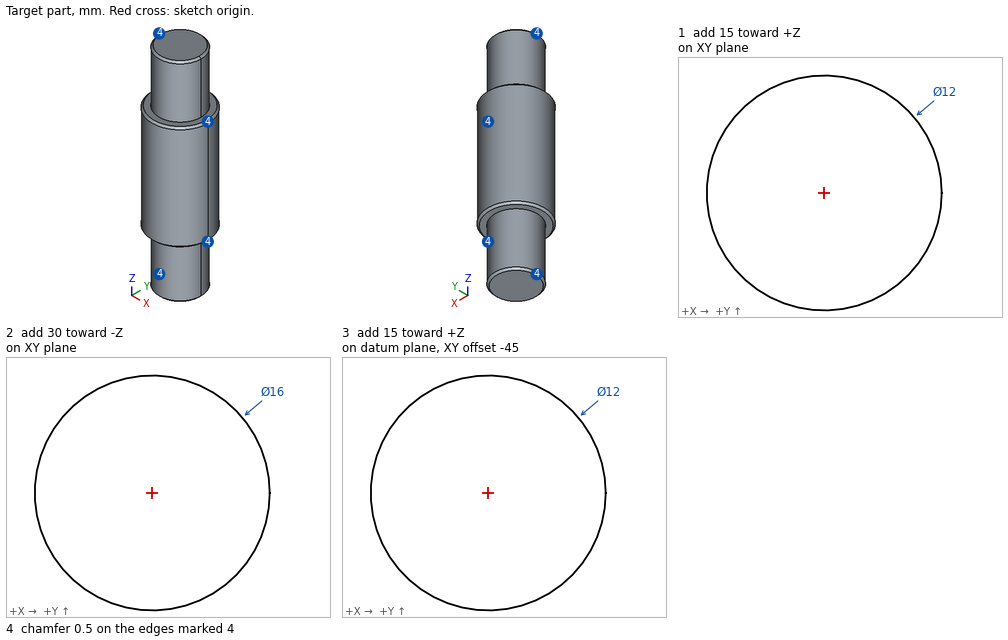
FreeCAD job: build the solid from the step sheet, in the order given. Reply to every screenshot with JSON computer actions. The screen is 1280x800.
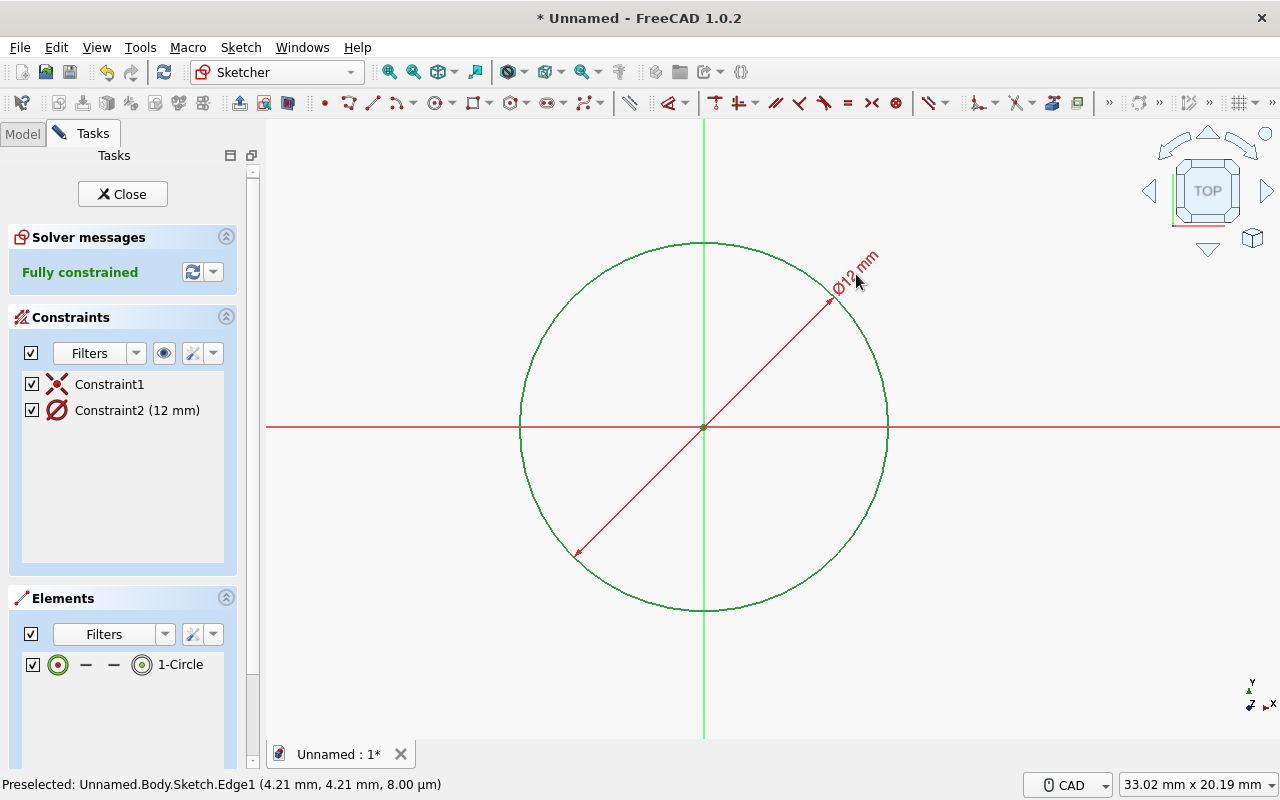
{"action": "left_click", "coordinate": [123, 194]}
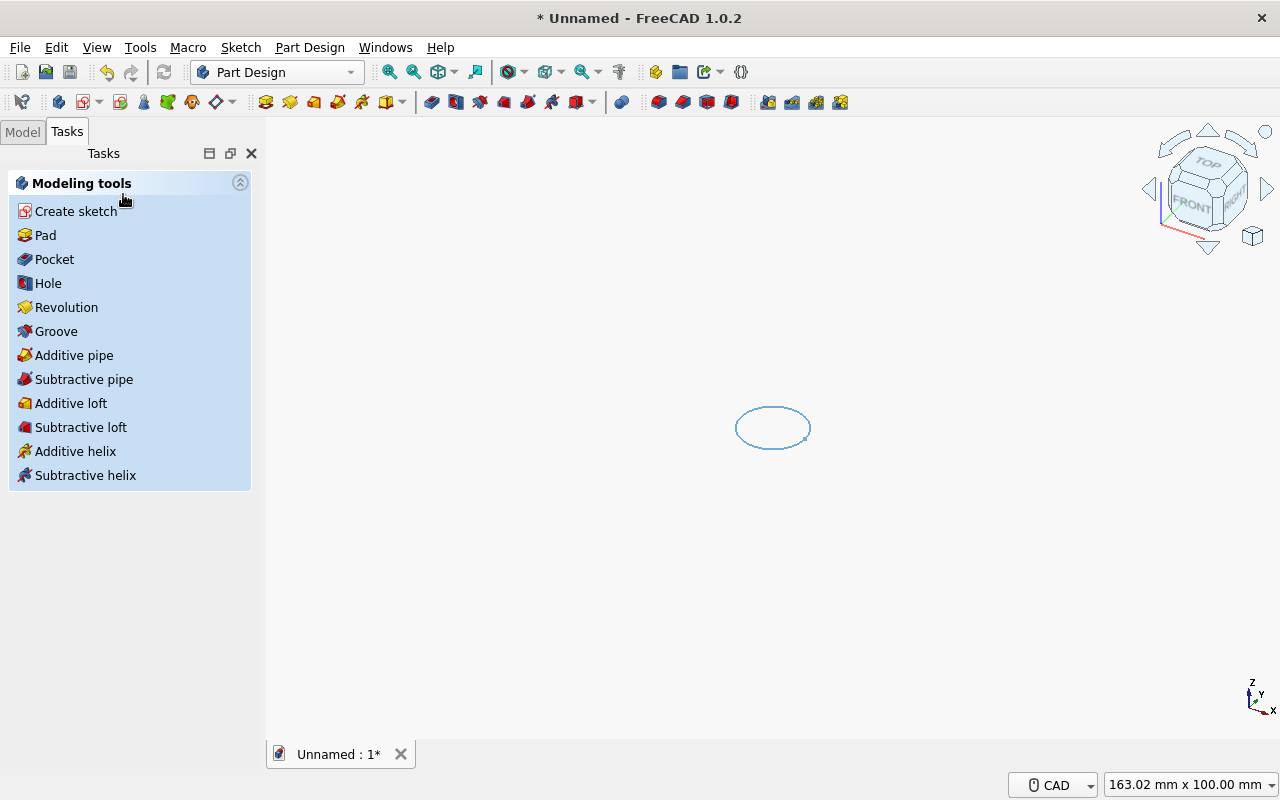
{"action": "left_click", "coordinate": [266, 102]}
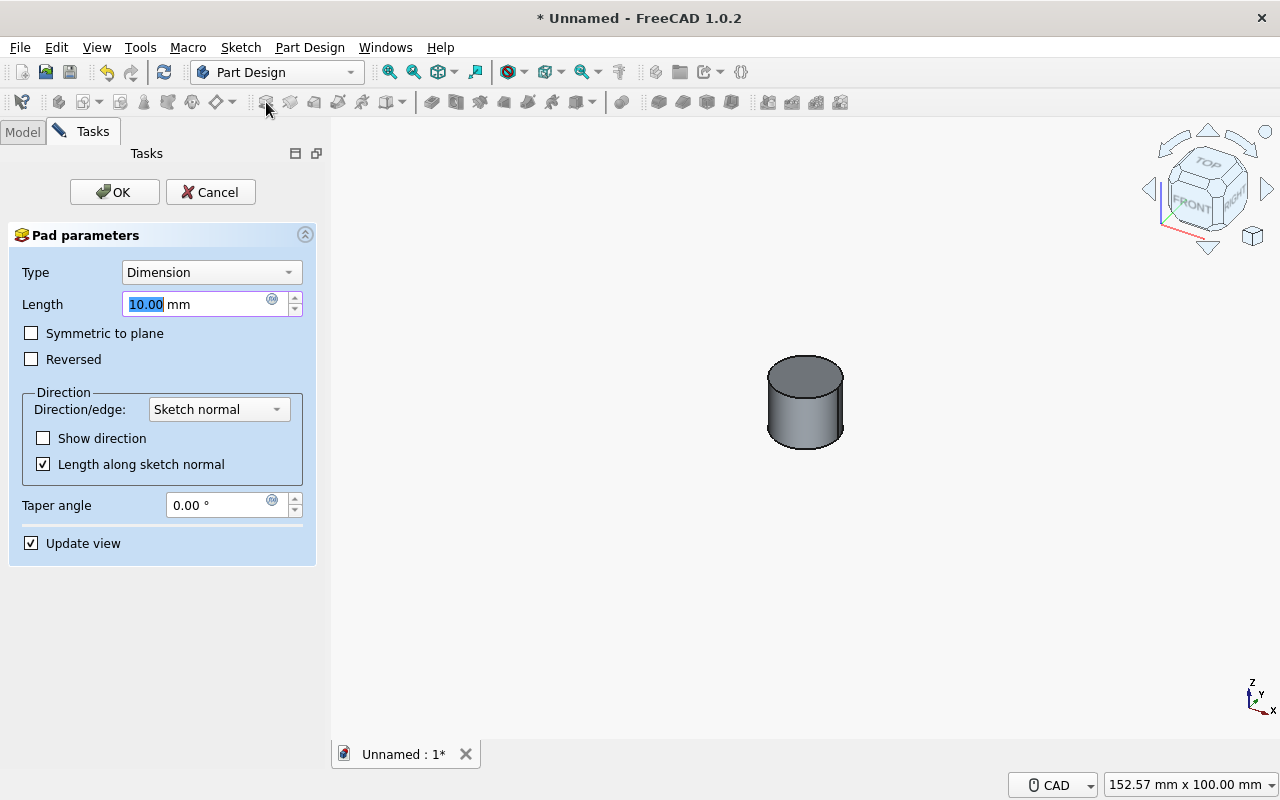
{"action": "type", "text": "15"}
{"action": "key", "text": "Tab"}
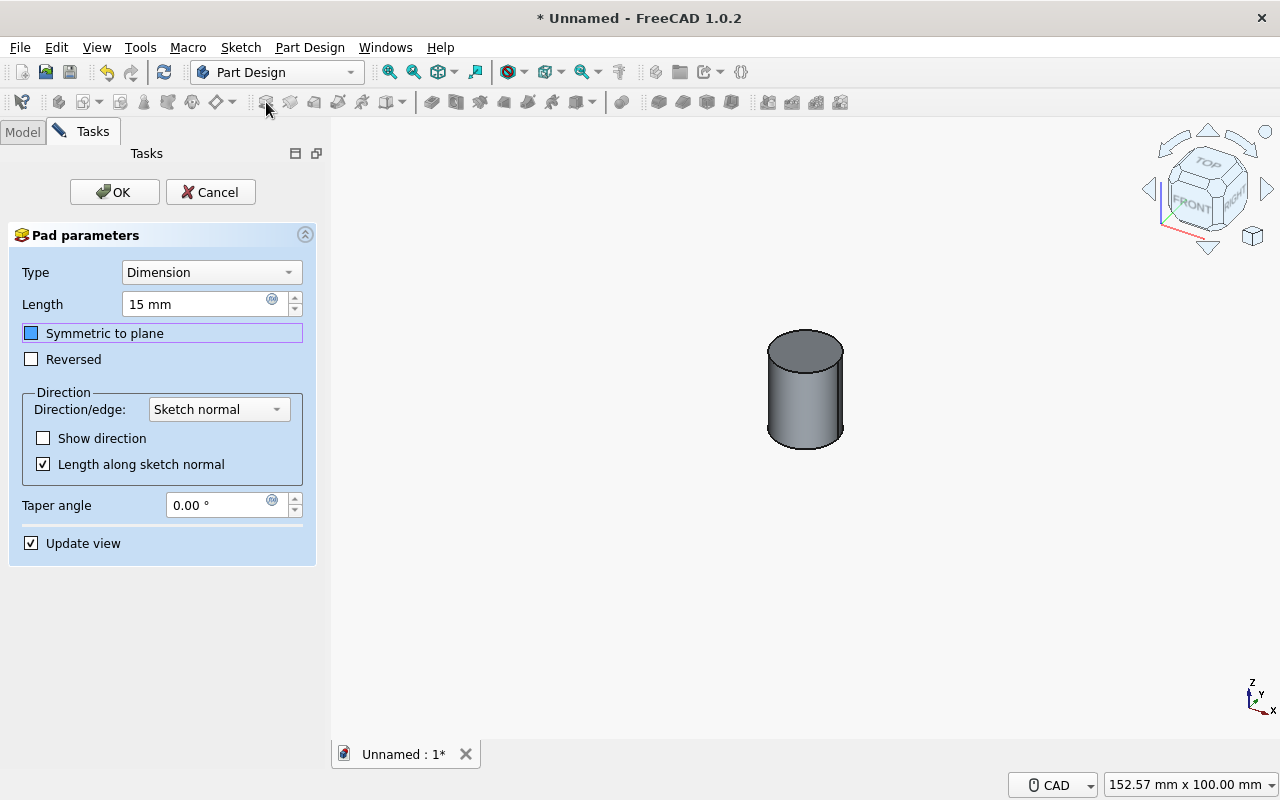
{"action": "left_click", "coordinate": [115, 192]}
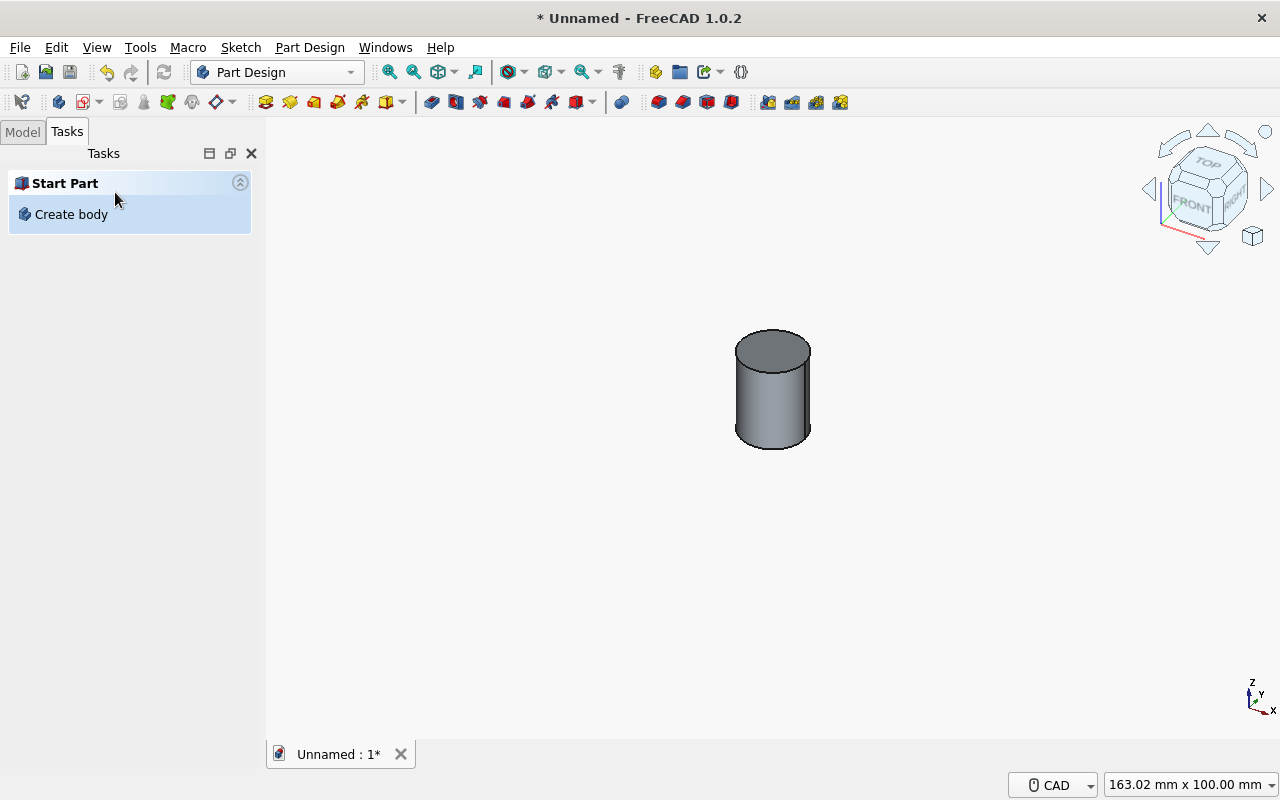
{"action": "left_click", "coordinate": [390, 72]}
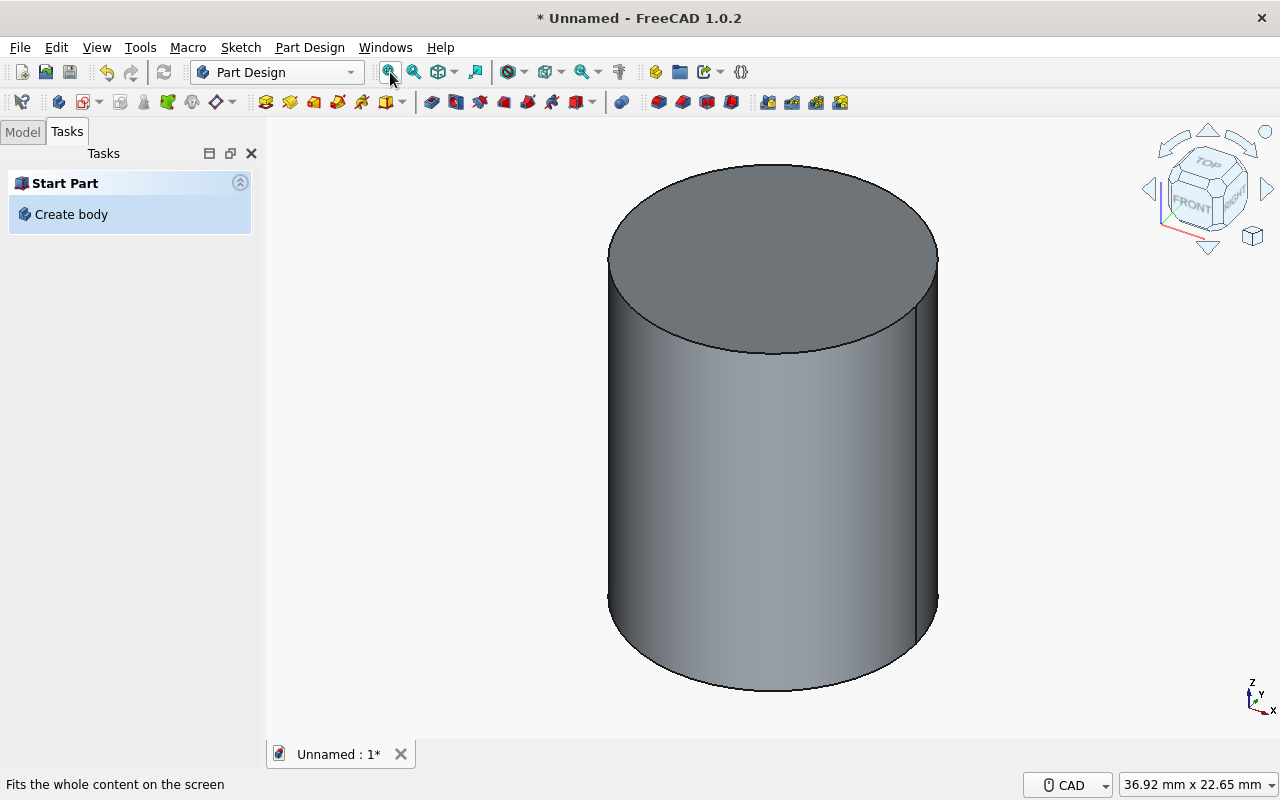
{"action": "left_click", "coordinate": [84, 102]}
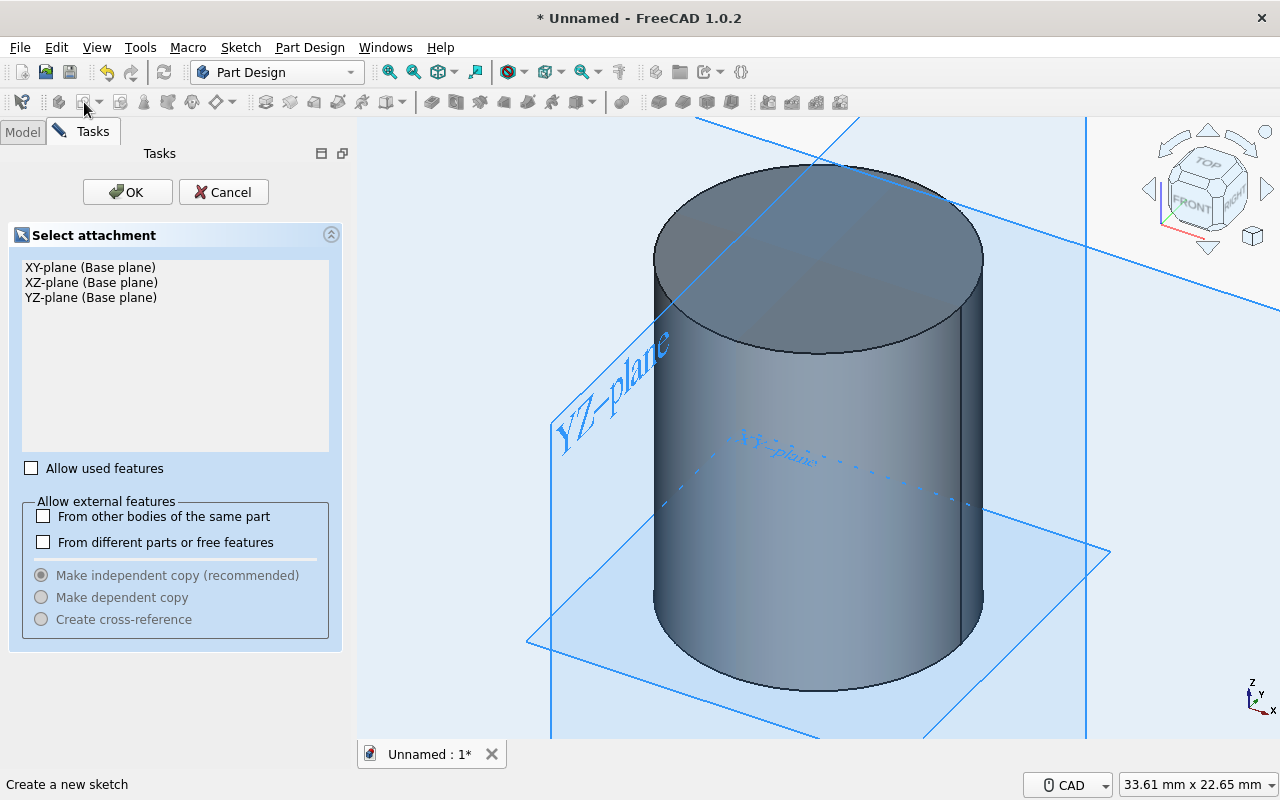
{"action": "left_click", "coordinate": [82, 268]}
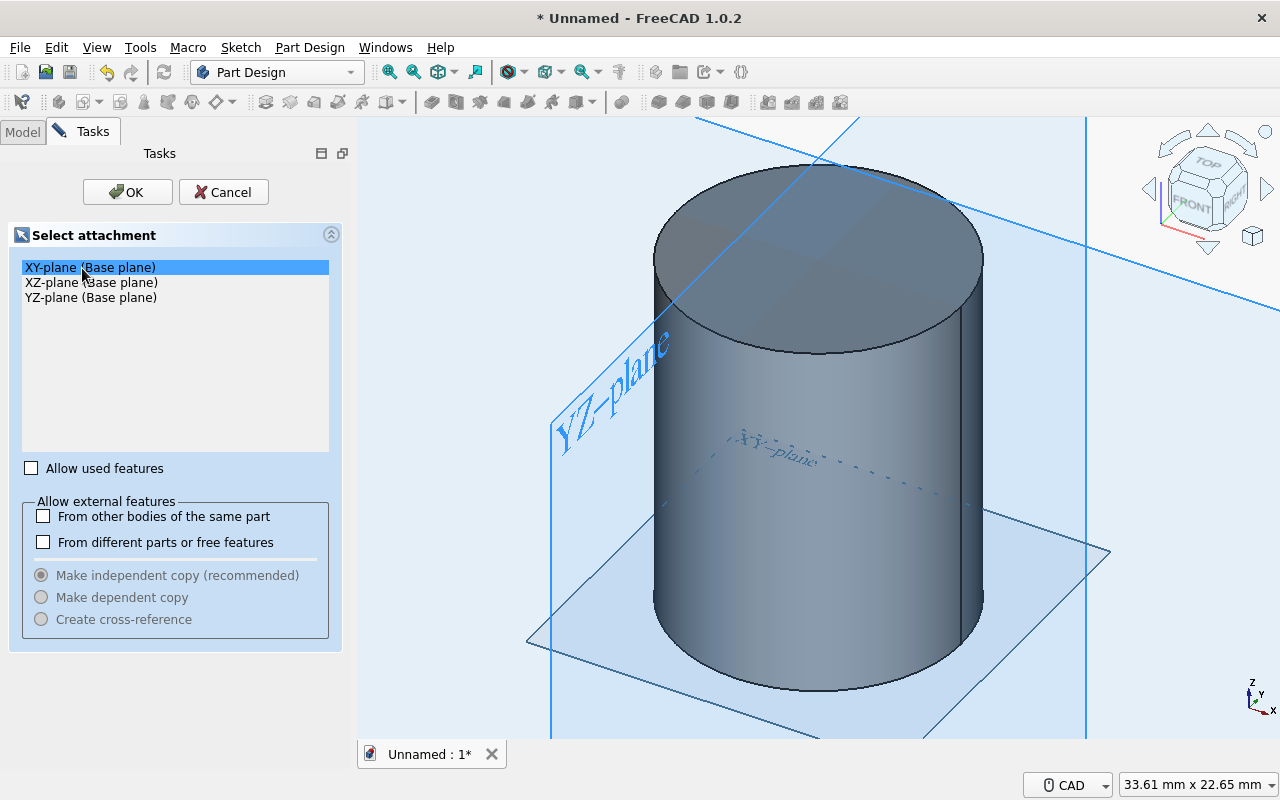
{"action": "left_click", "coordinate": [128, 192]}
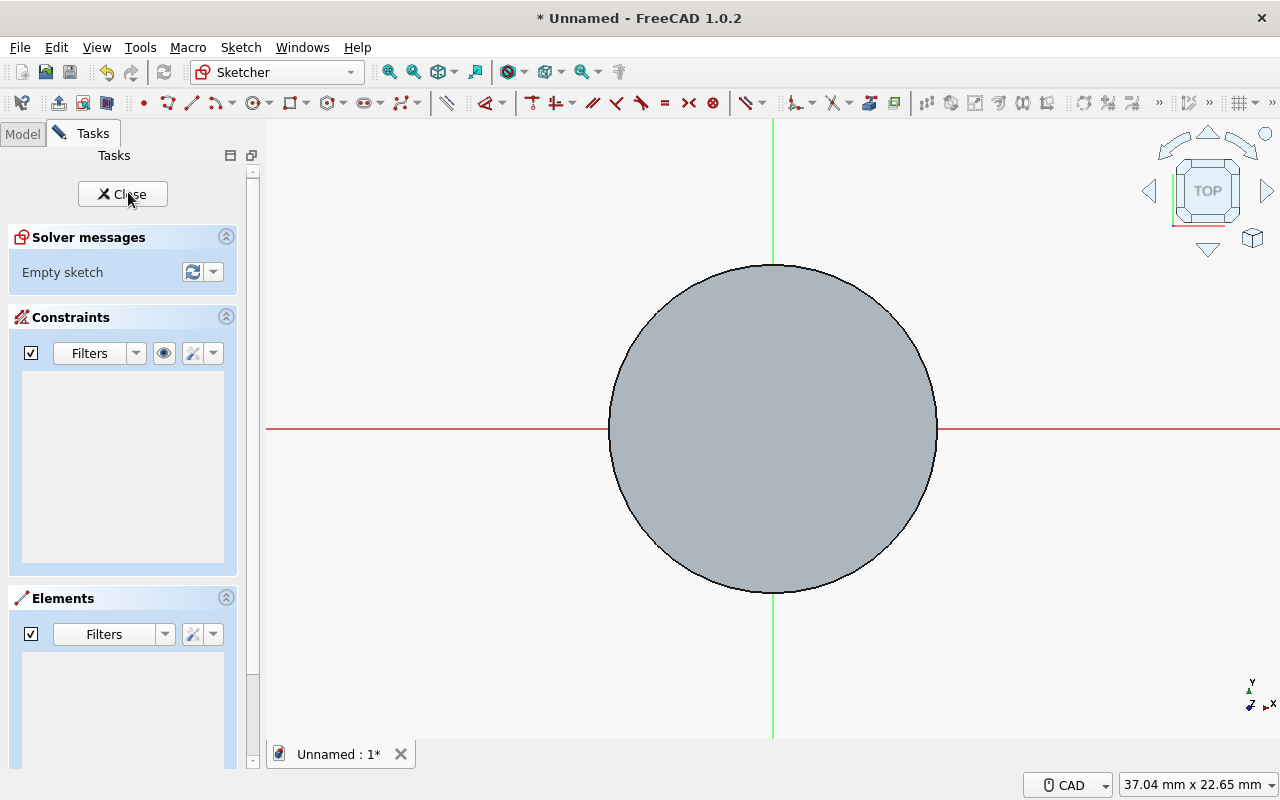
{"action": "left_click", "coordinate": [108, 104]}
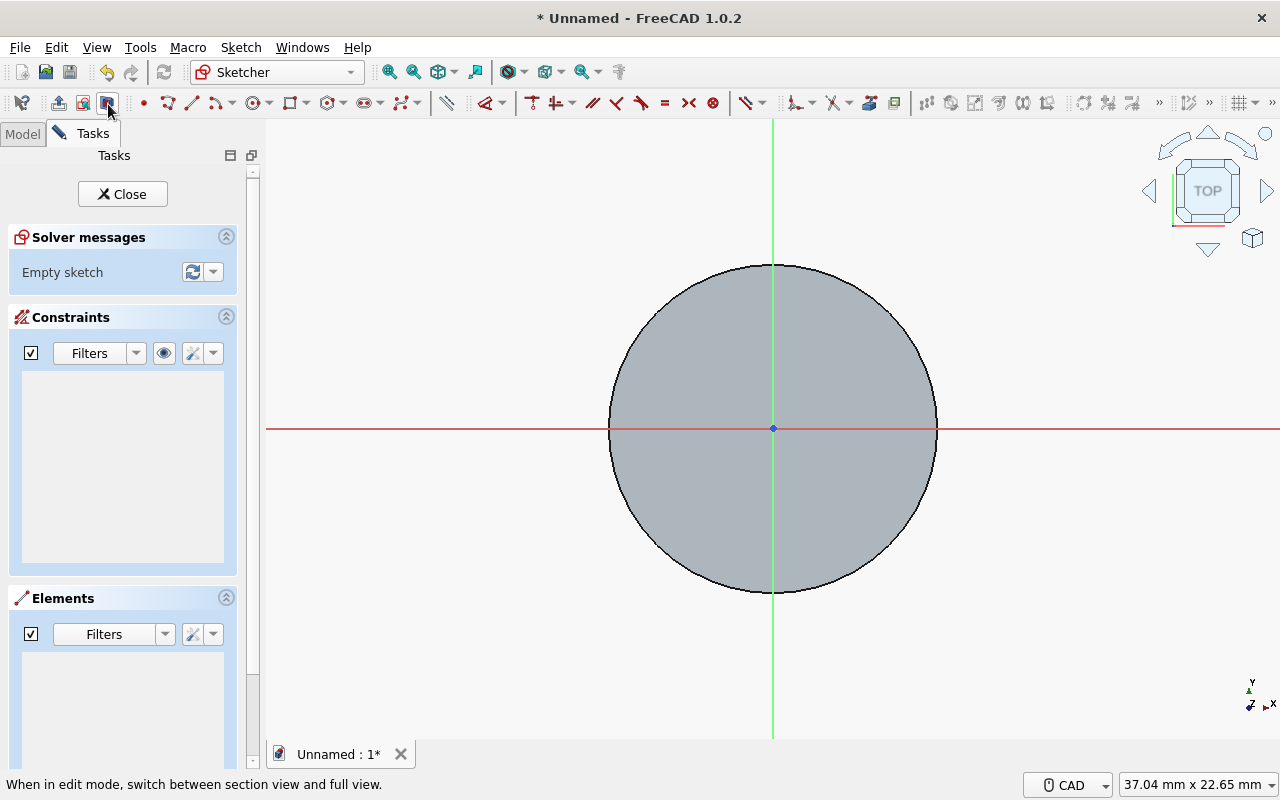
{"action": "left_click", "coordinate": [254, 104]}